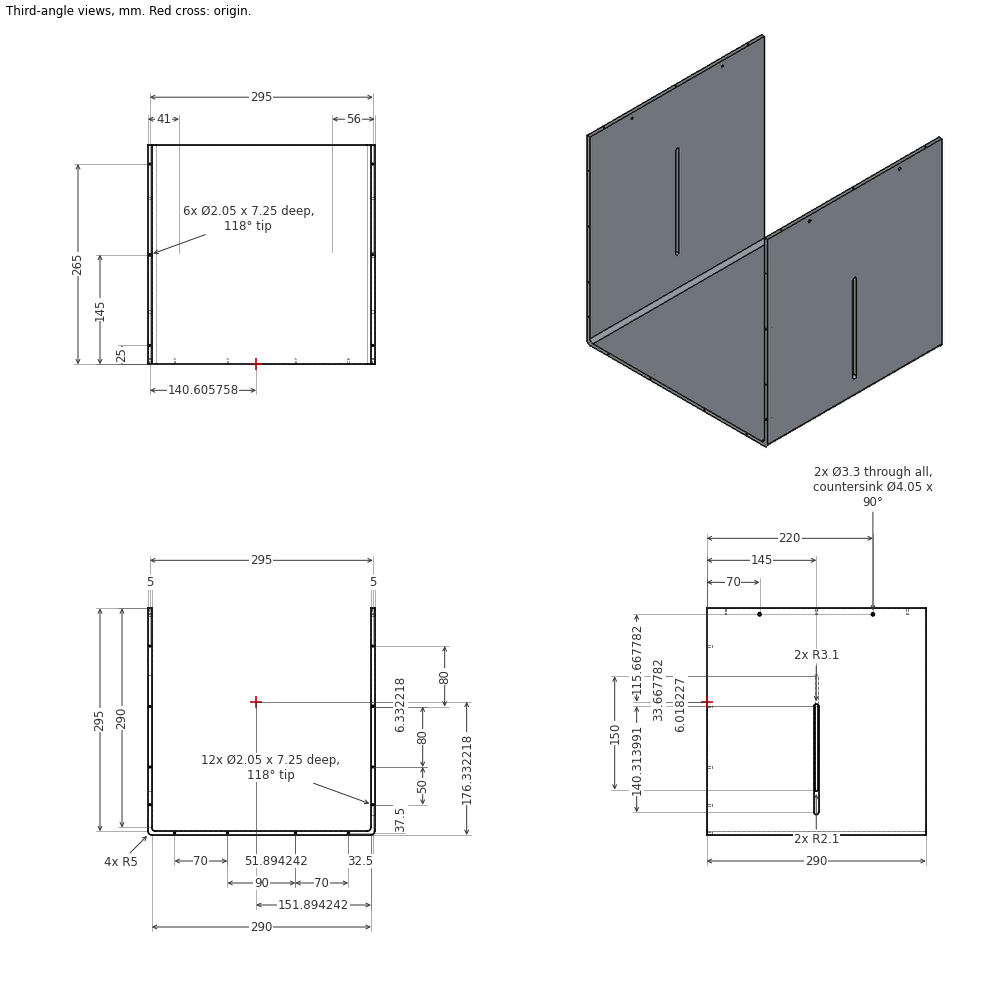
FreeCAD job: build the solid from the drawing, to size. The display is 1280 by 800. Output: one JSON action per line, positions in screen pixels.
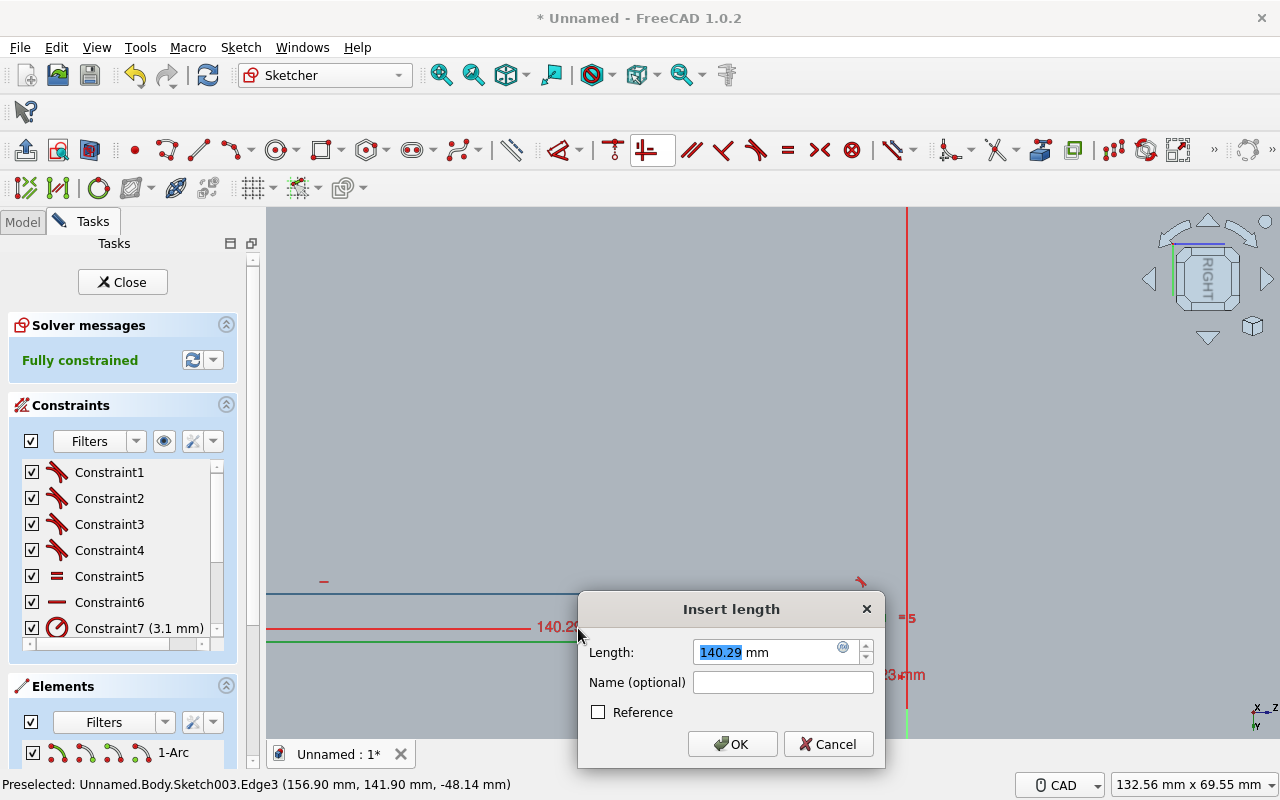
{"action": "type", "text": "140.313991"}
{"action": "key", "text": "Return"}
{"action": "key", "text": "Escape"}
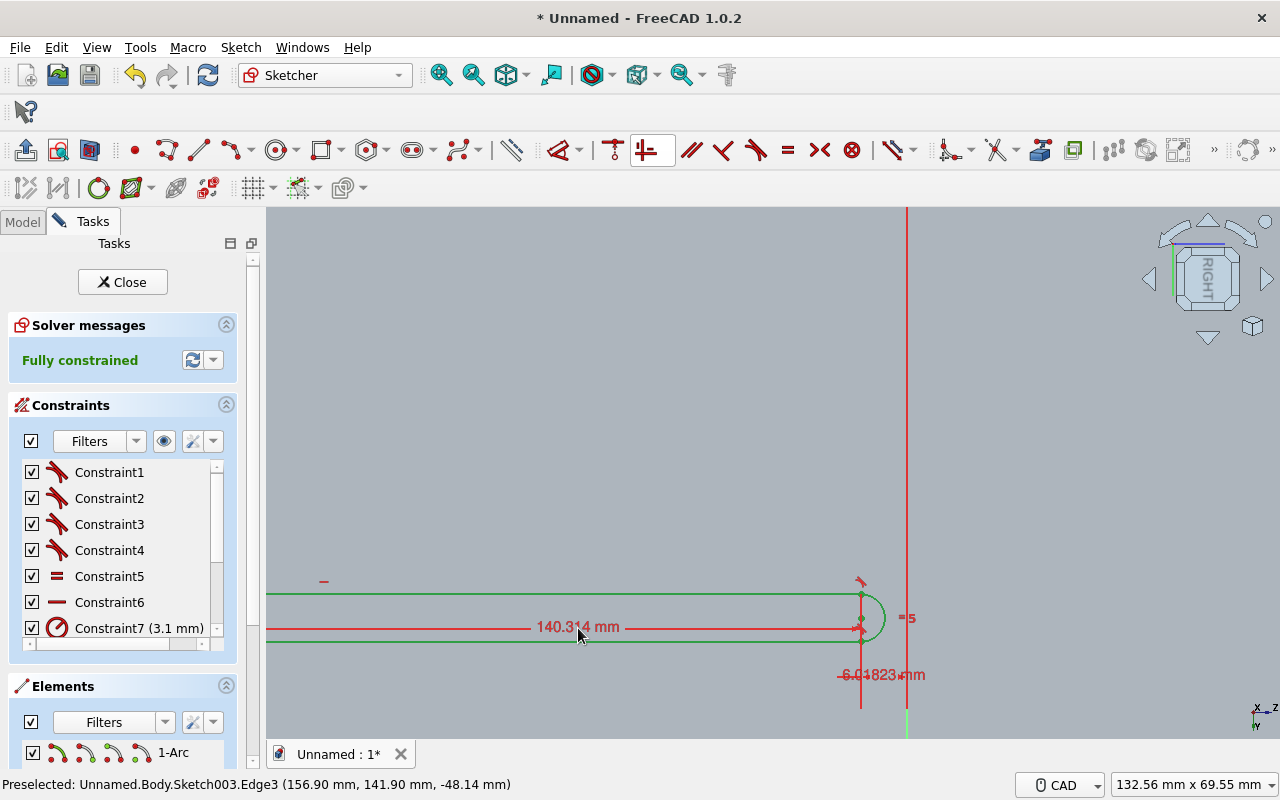
{"action": "left_click", "coordinate": [123, 282]}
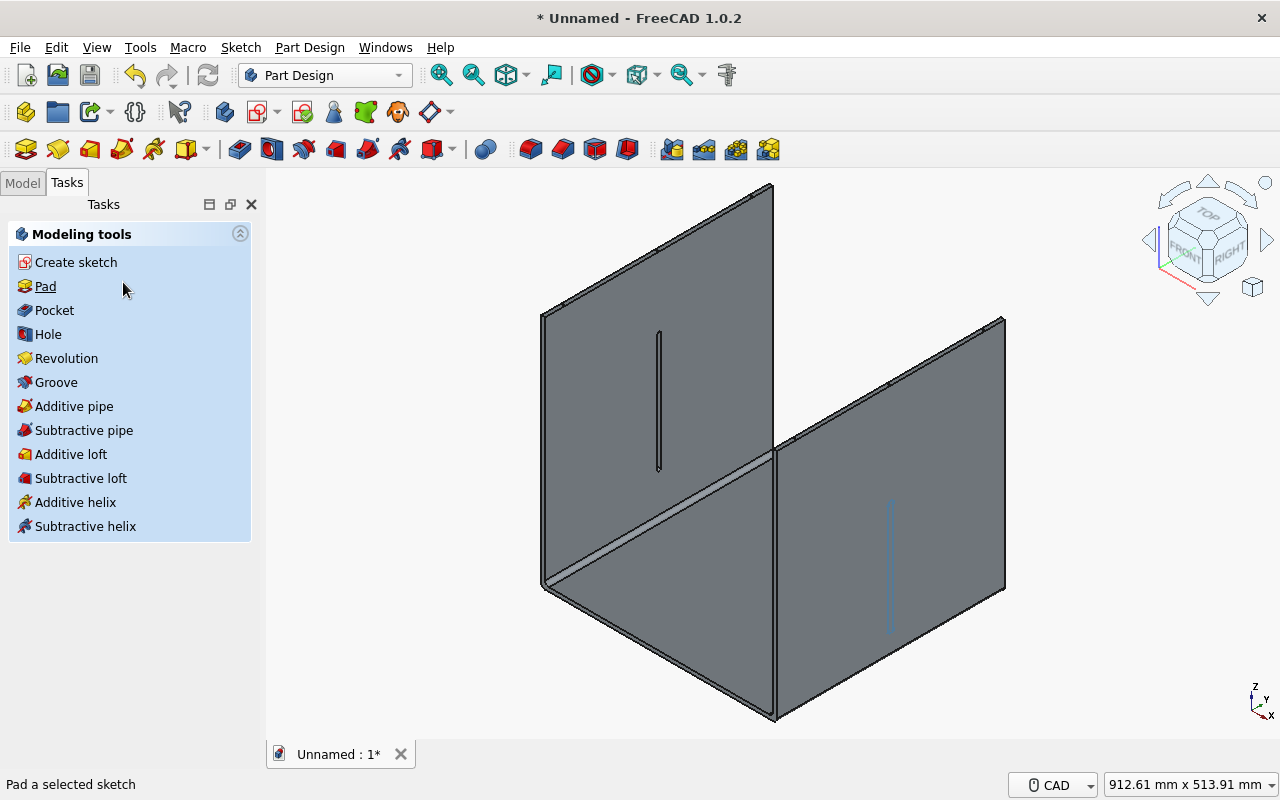
{"action": "left_click", "coordinate": [240, 150]}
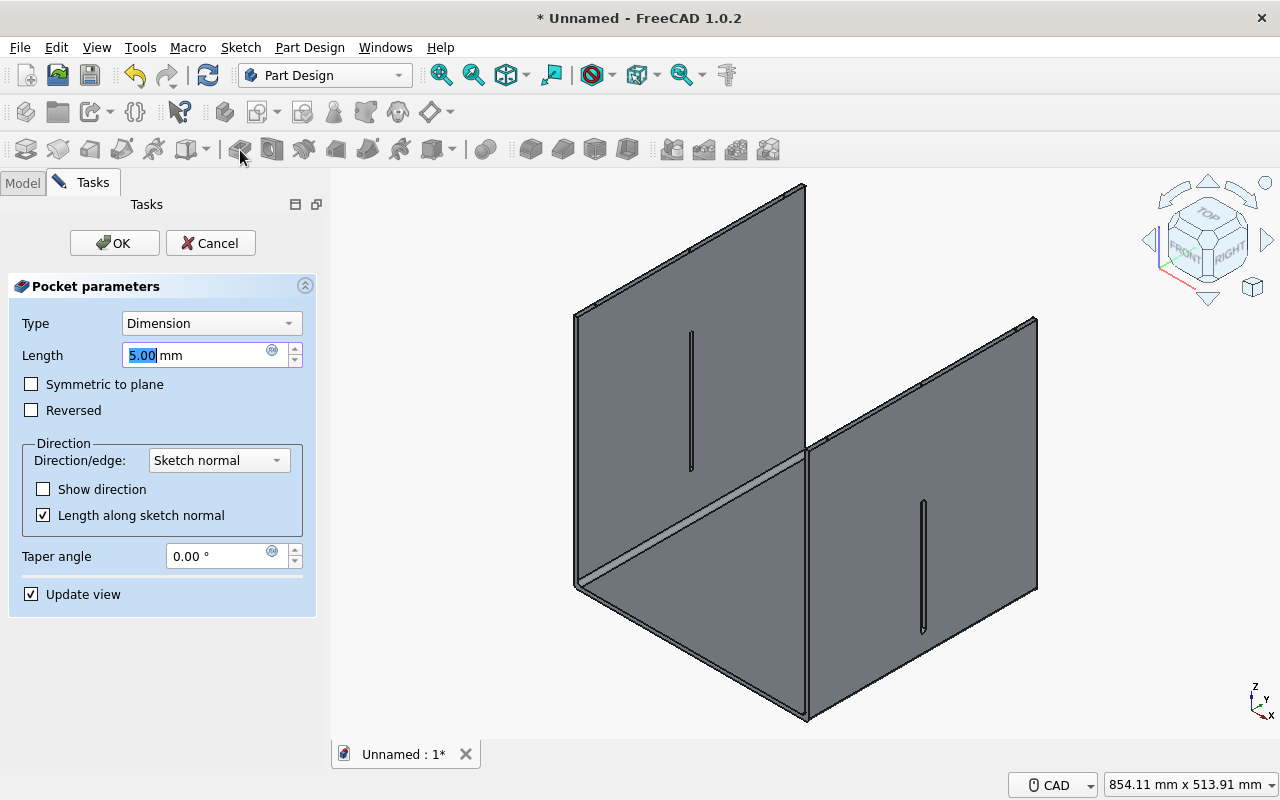
{"action": "type", "text": "56"}
{"action": "key", "text": "Tab"}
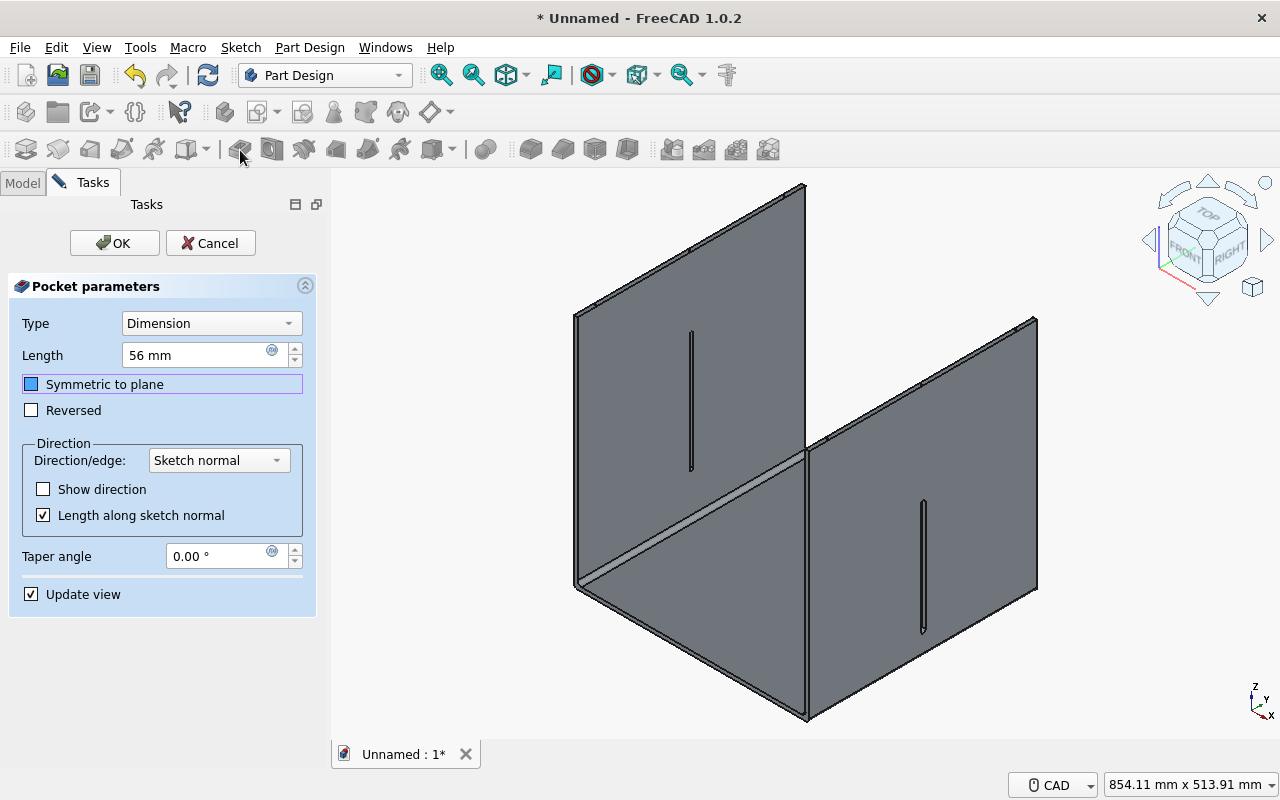
{"action": "left_click", "coordinate": [115, 243]}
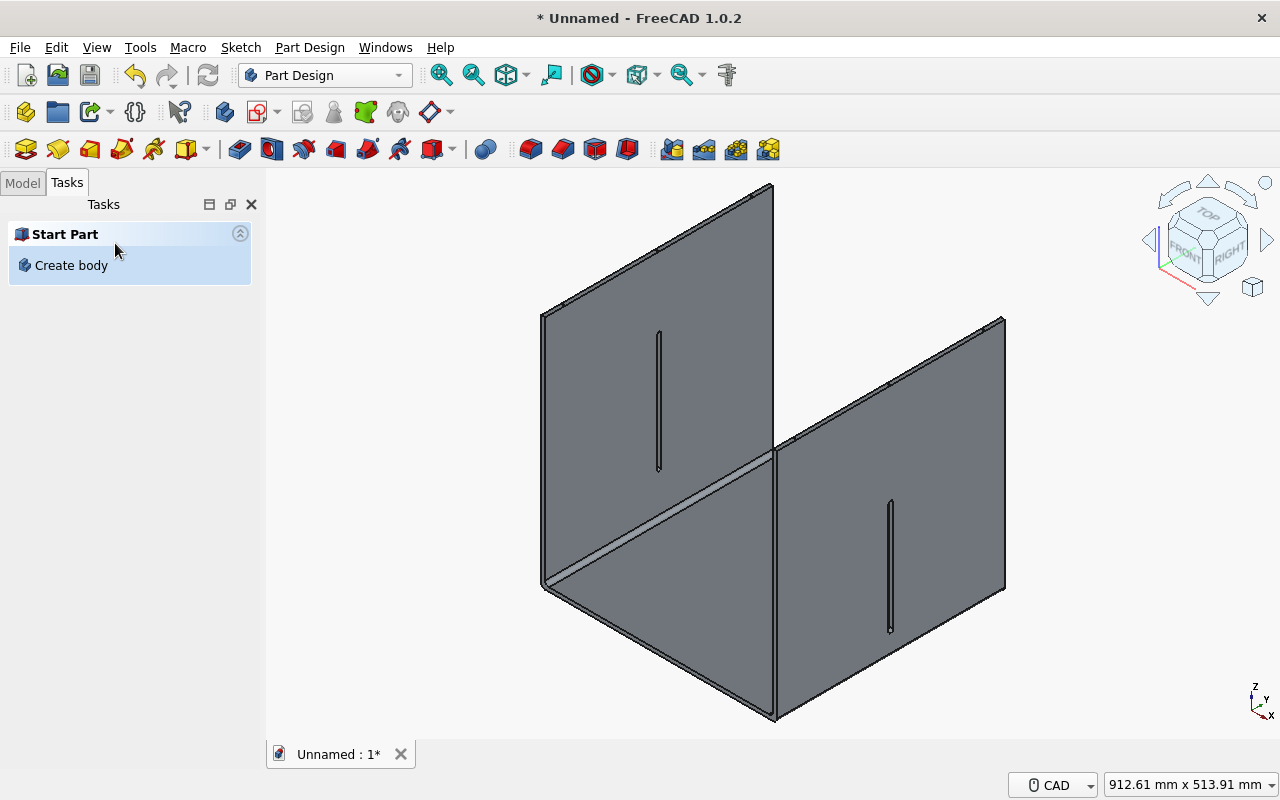
{"action": "left_click", "coordinate": [923, 423]}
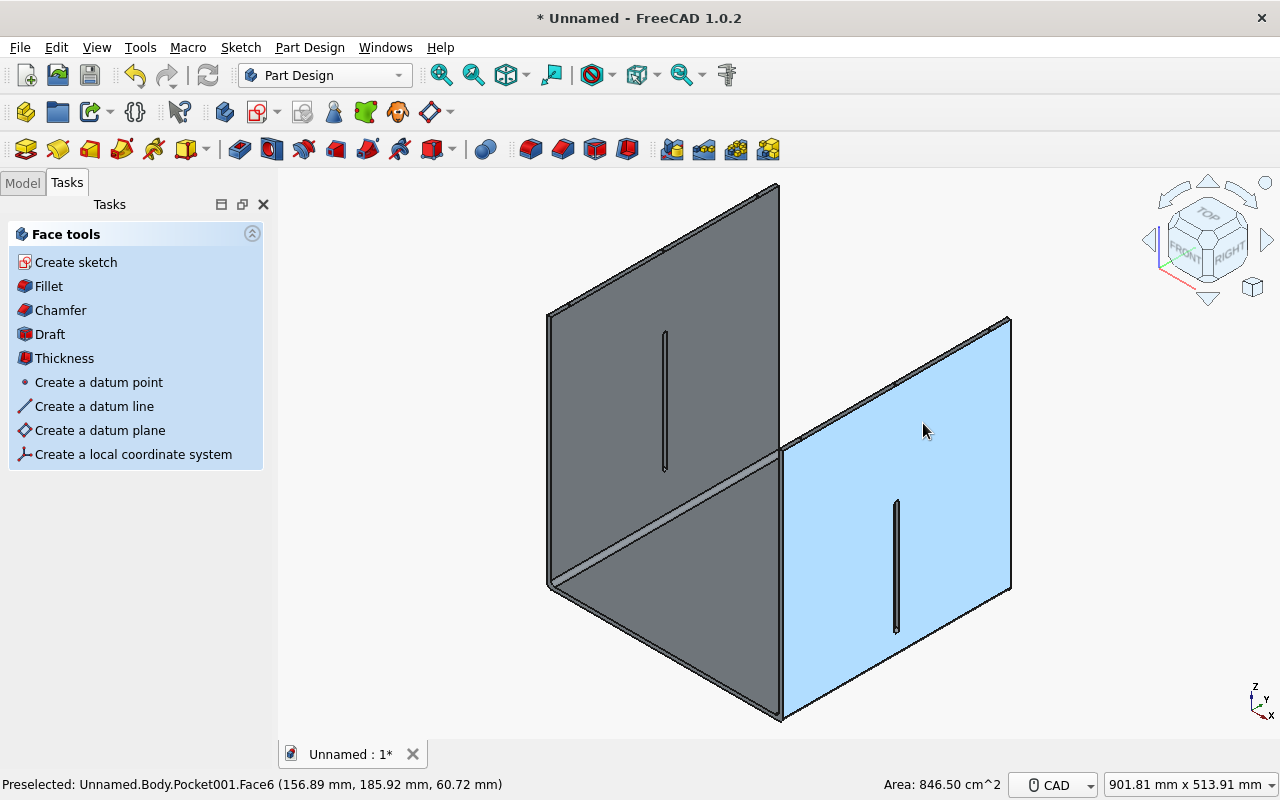
{"action": "left_click", "coordinate": [258, 112]}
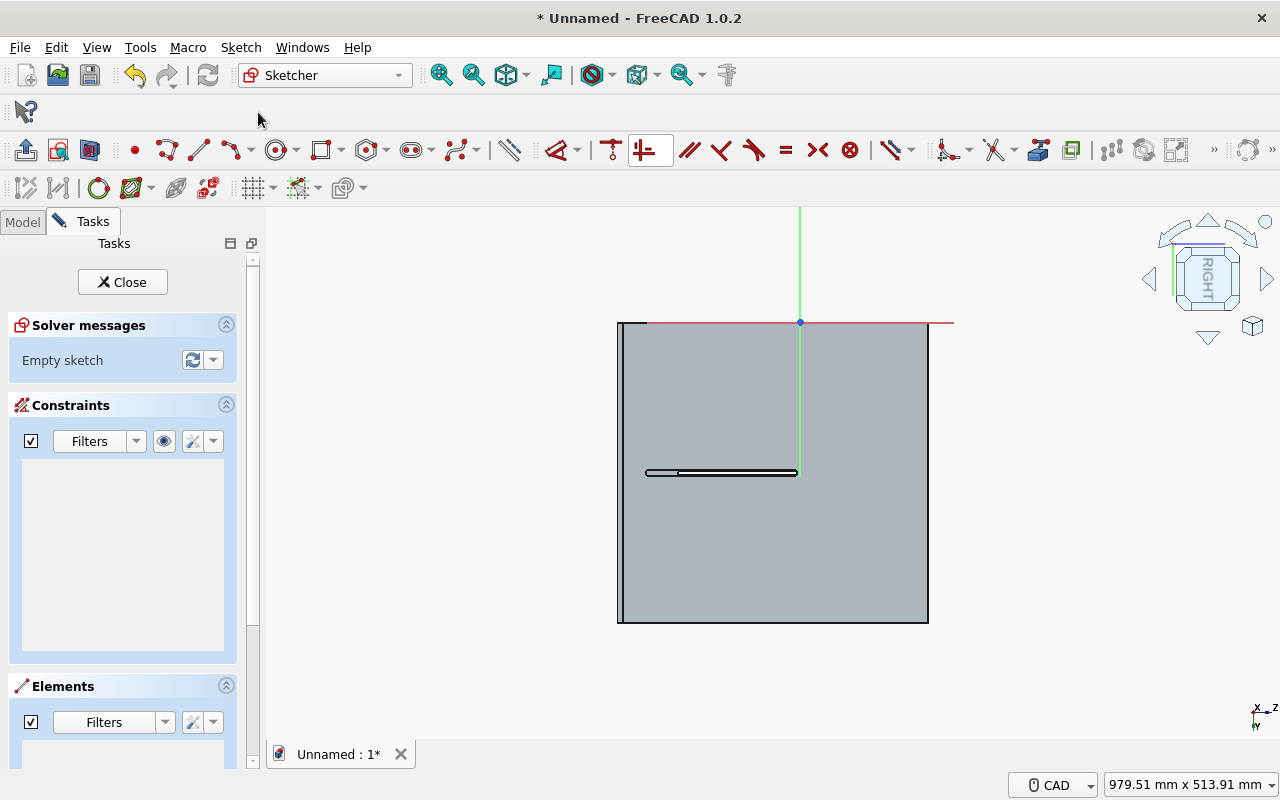
{"action": "scroll", "coordinate": [1115, 366], "scroll_direction": "up", "scroll_amount": 2}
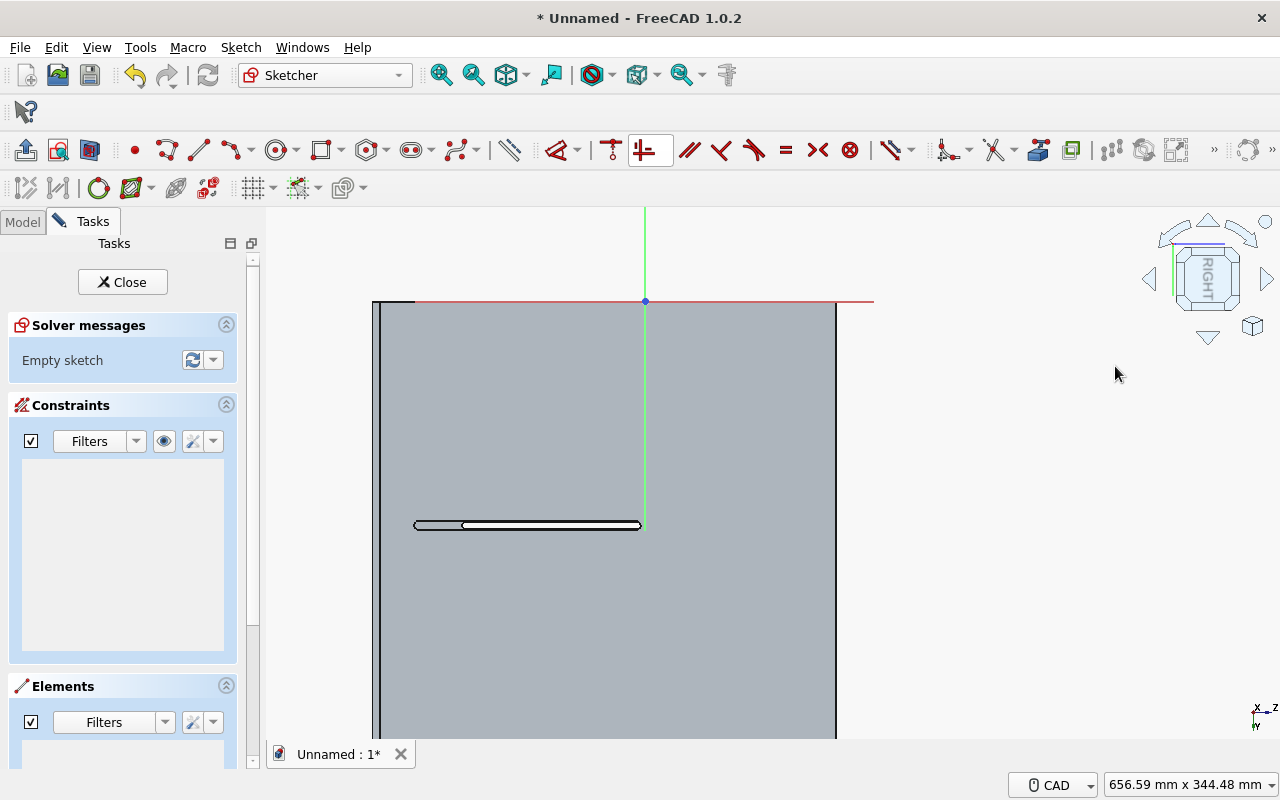
{"action": "left_click", "coordinate": [276, 150]}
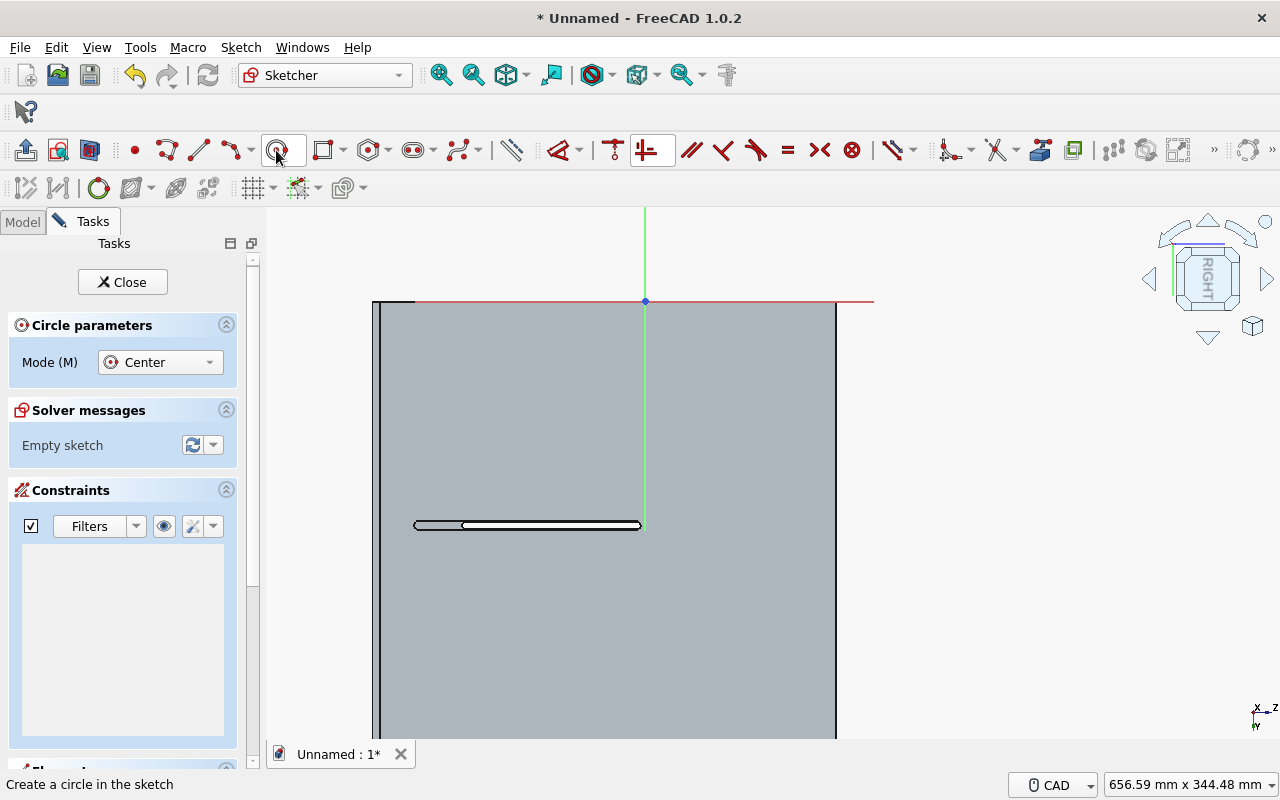
{"action": "scroll", "coordinate": [824, 641], "scroll_direction": "up", "scroll_amount": 11}